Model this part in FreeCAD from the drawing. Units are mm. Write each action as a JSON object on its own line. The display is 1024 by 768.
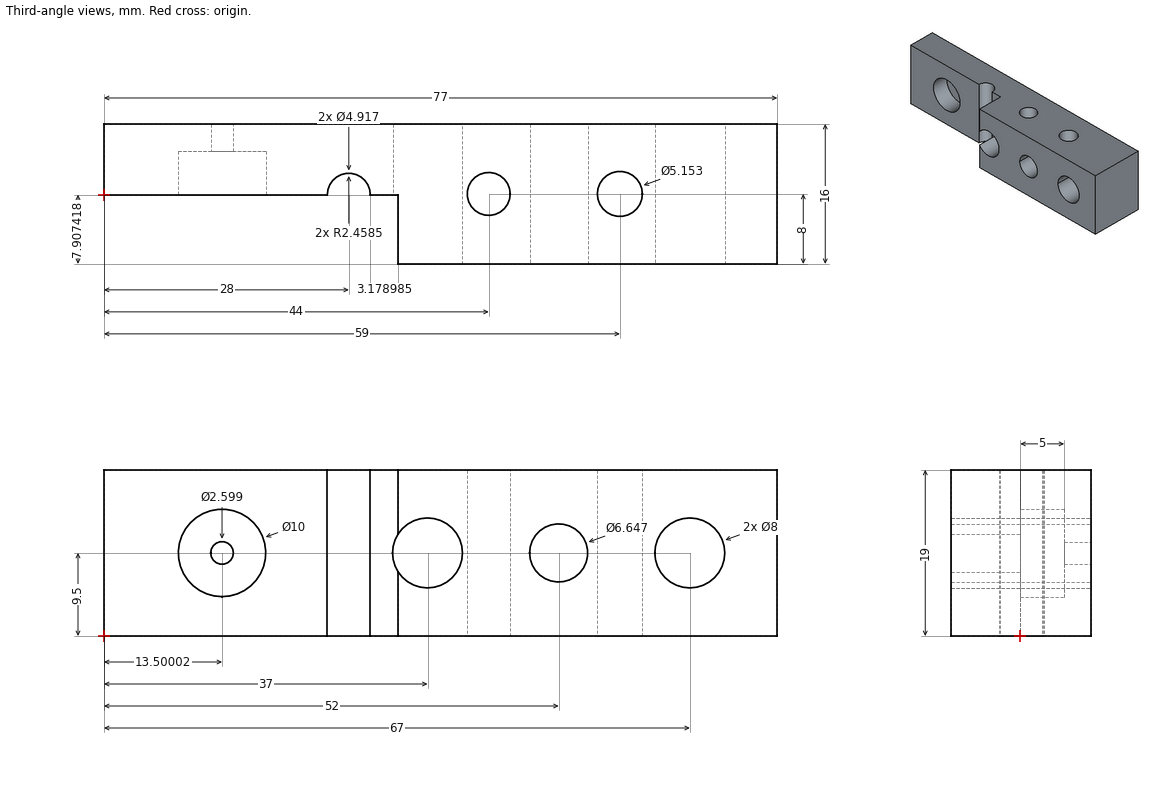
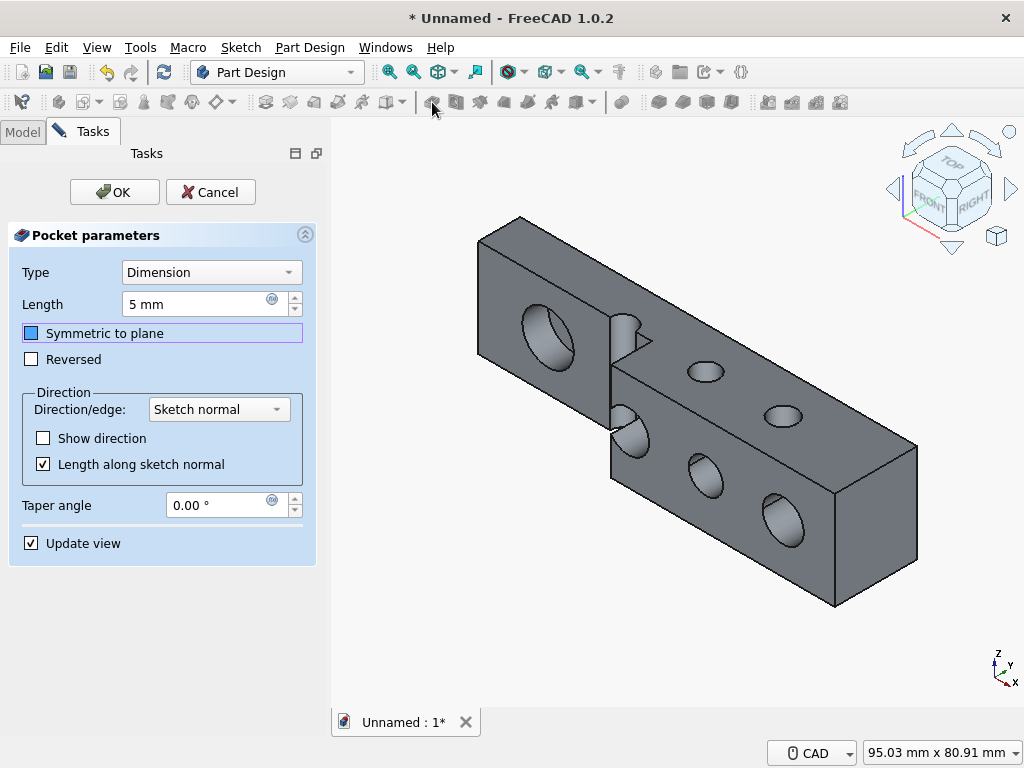
{"action": "left_click", "coordinate": [115, 192]}